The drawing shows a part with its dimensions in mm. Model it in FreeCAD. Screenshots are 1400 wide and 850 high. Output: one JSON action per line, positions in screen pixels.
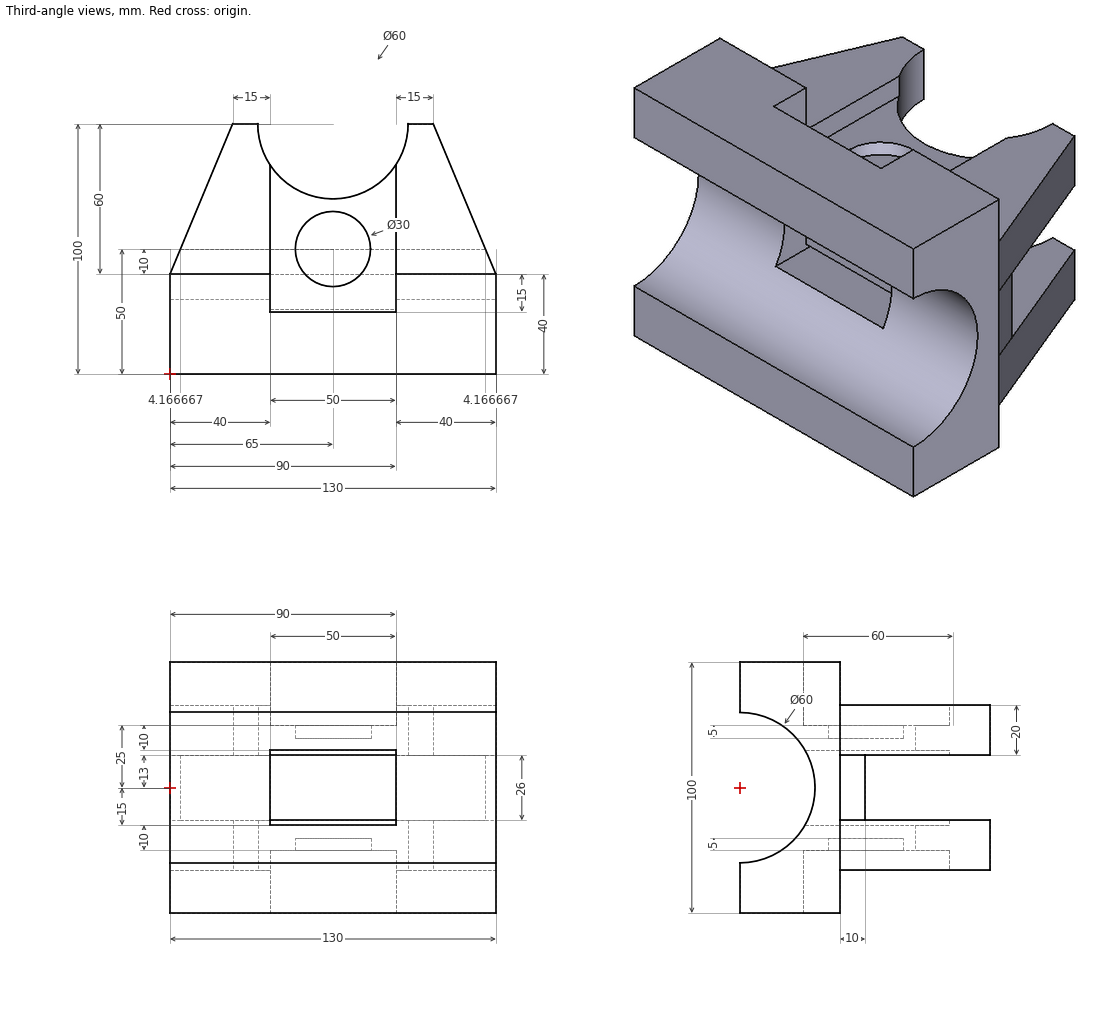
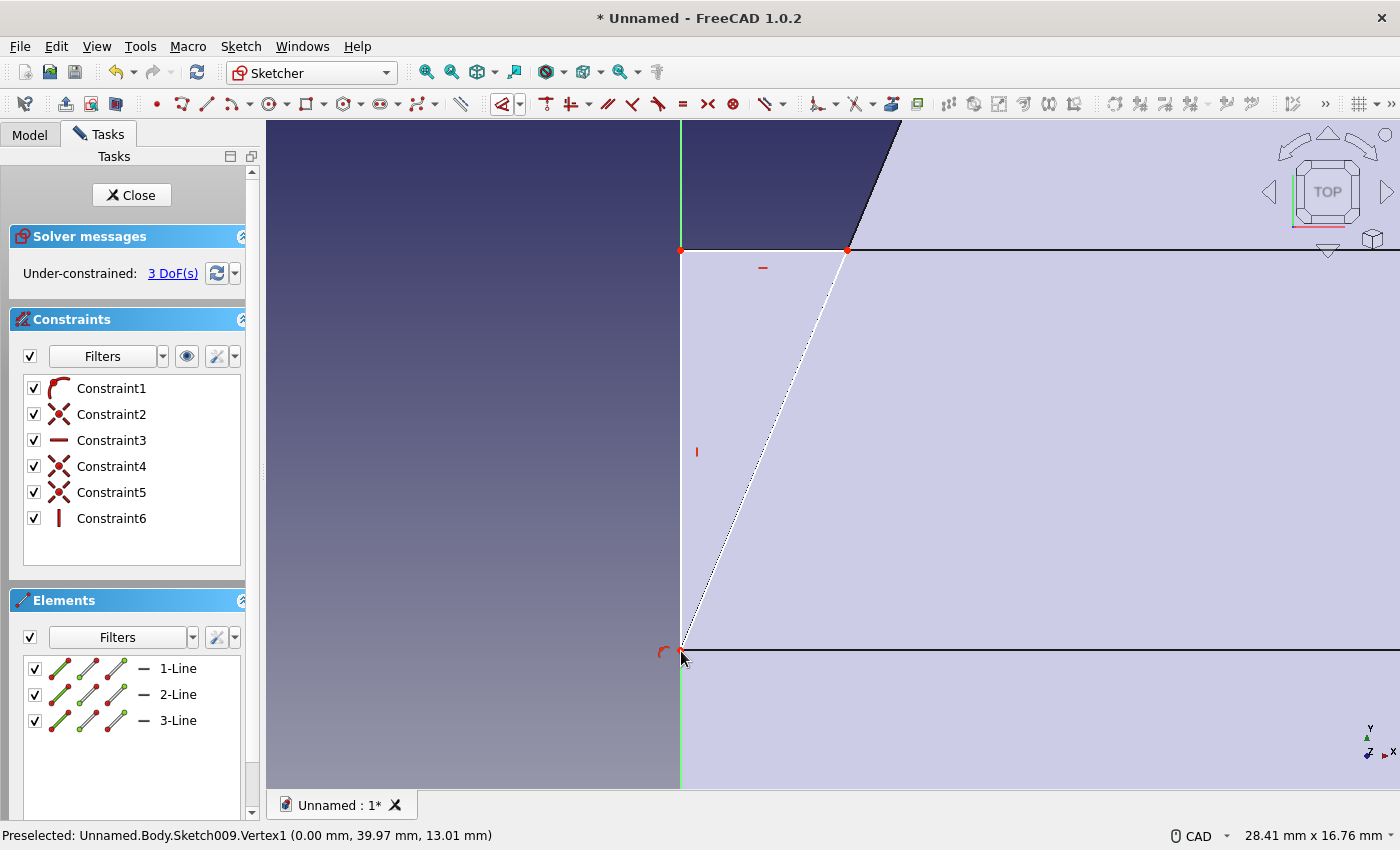
{"action": "left_click", "coordinate": [681, 371]}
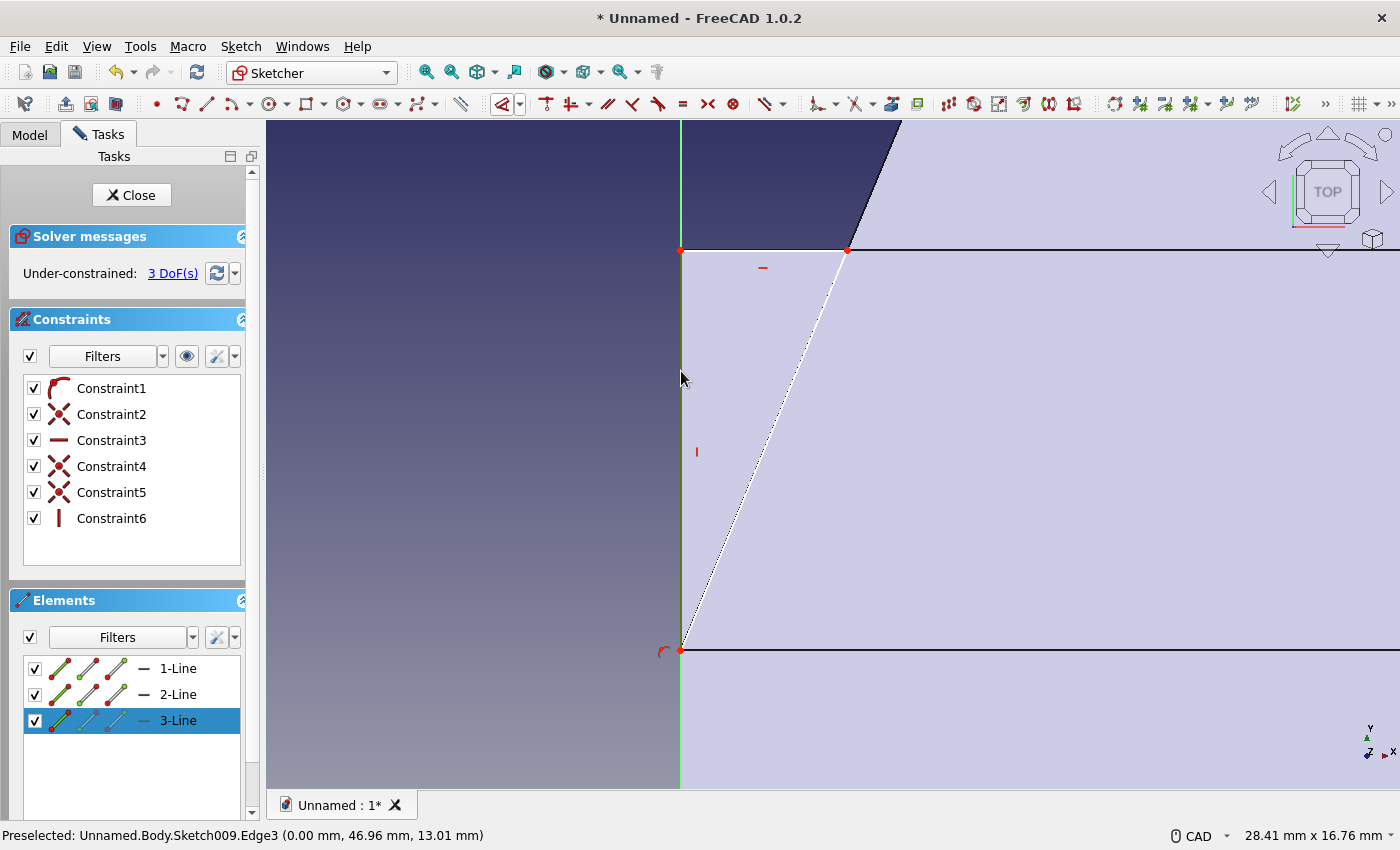
{"action": "key", "text": "i"}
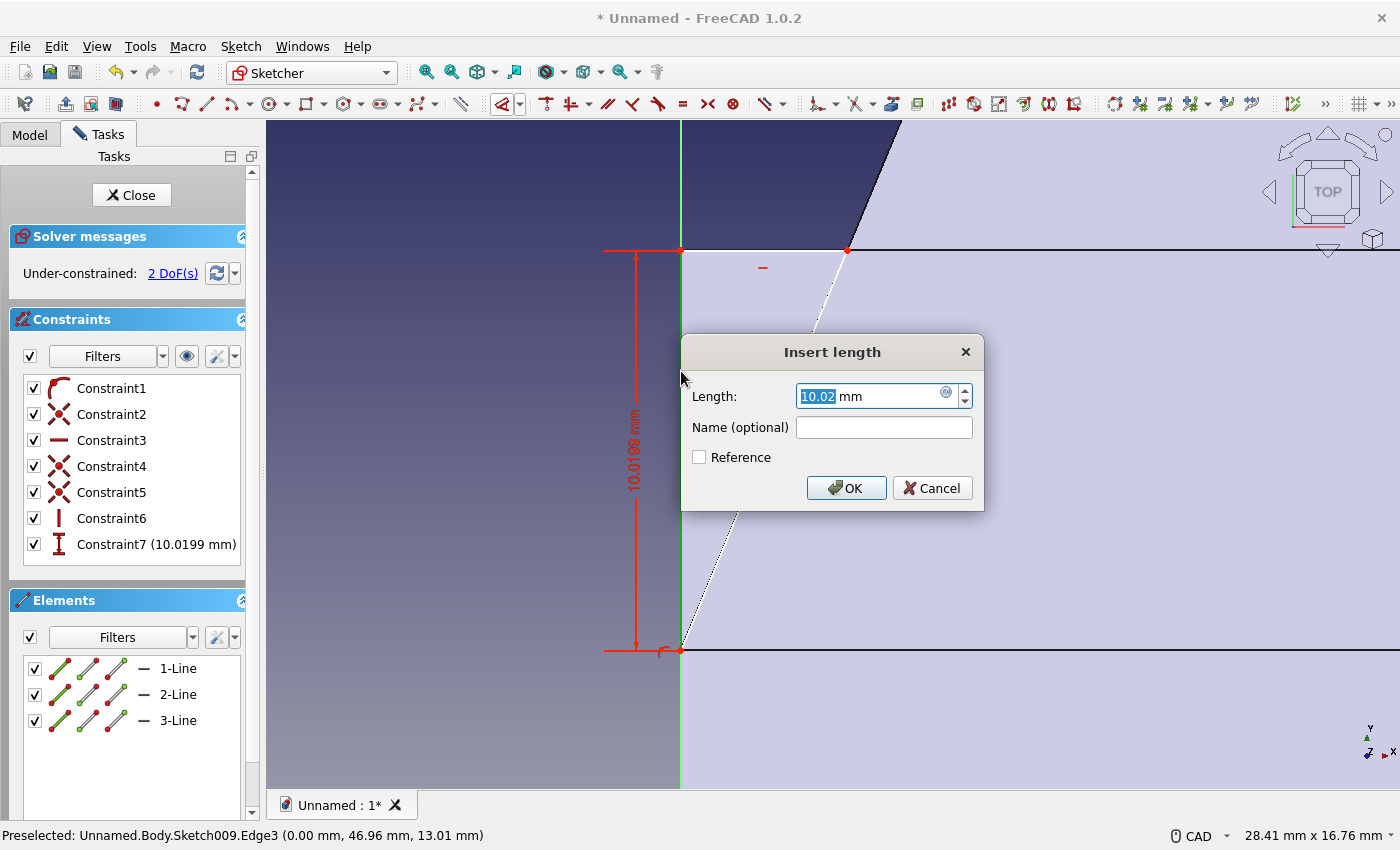
{"action": "type", "text": "10"}
{"action": "key", "text": "Return"}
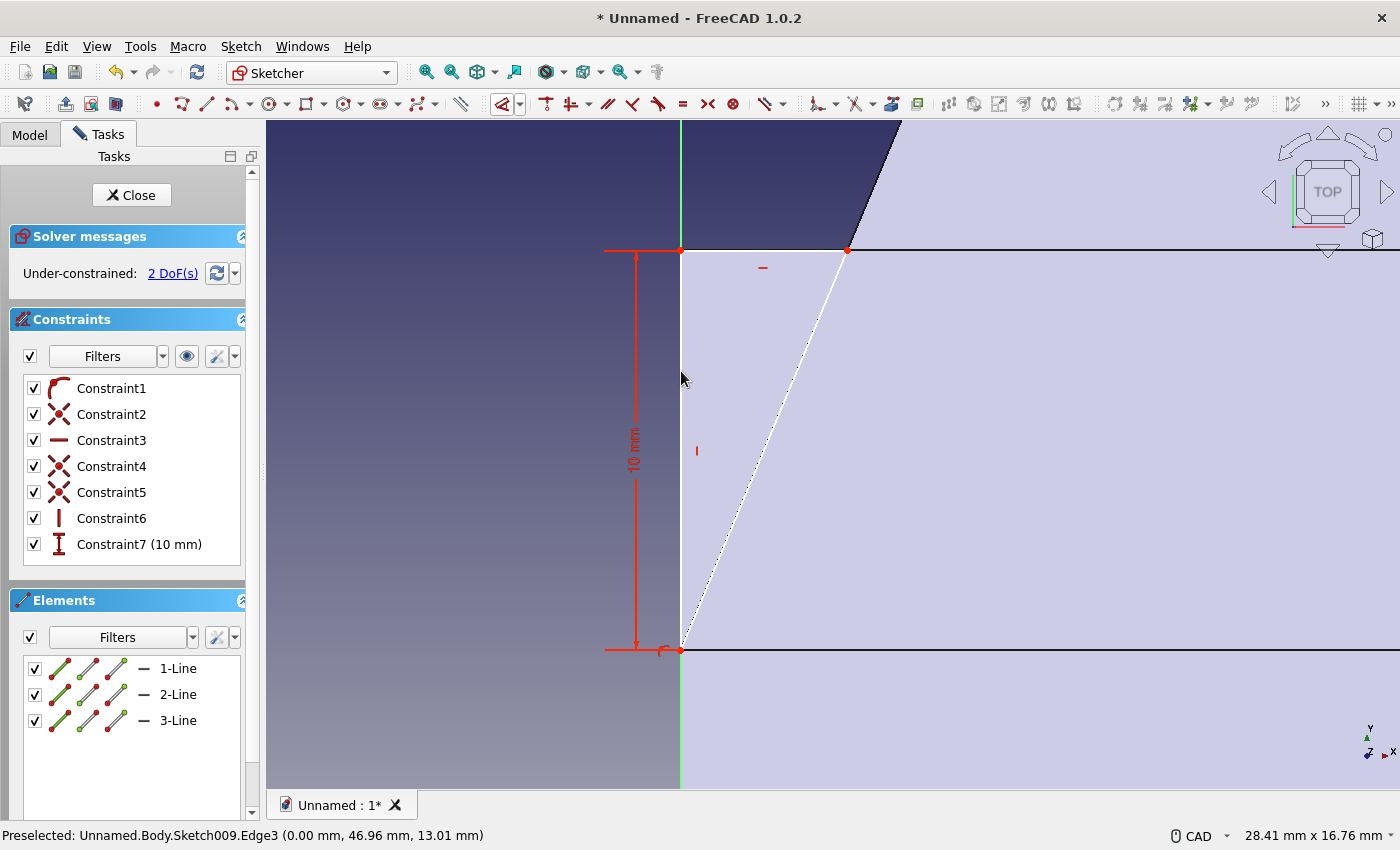
{"action": "left_click", "coordinate": [681, 650]}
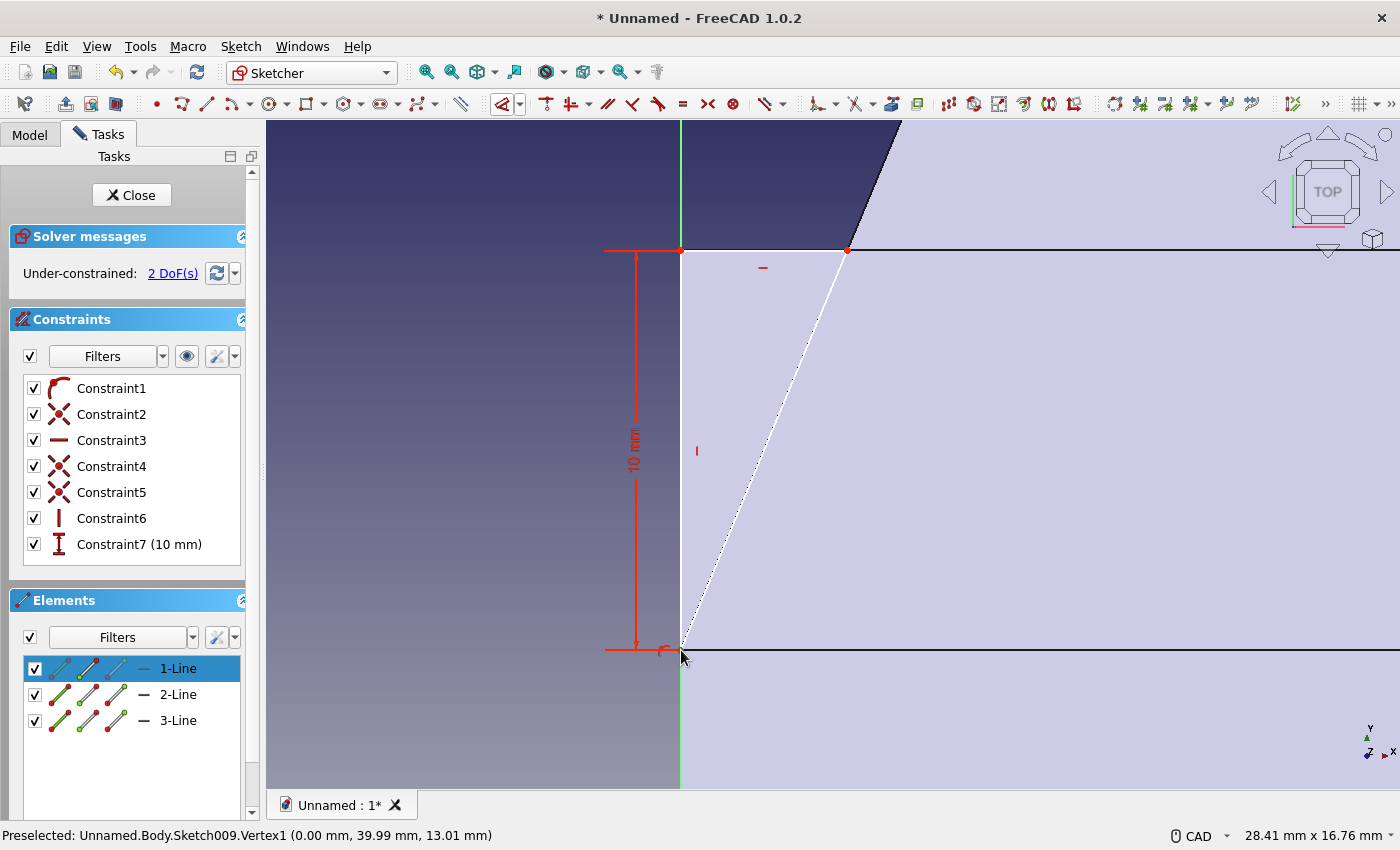
{"action": "left_click", "coordinate": [520, 104]}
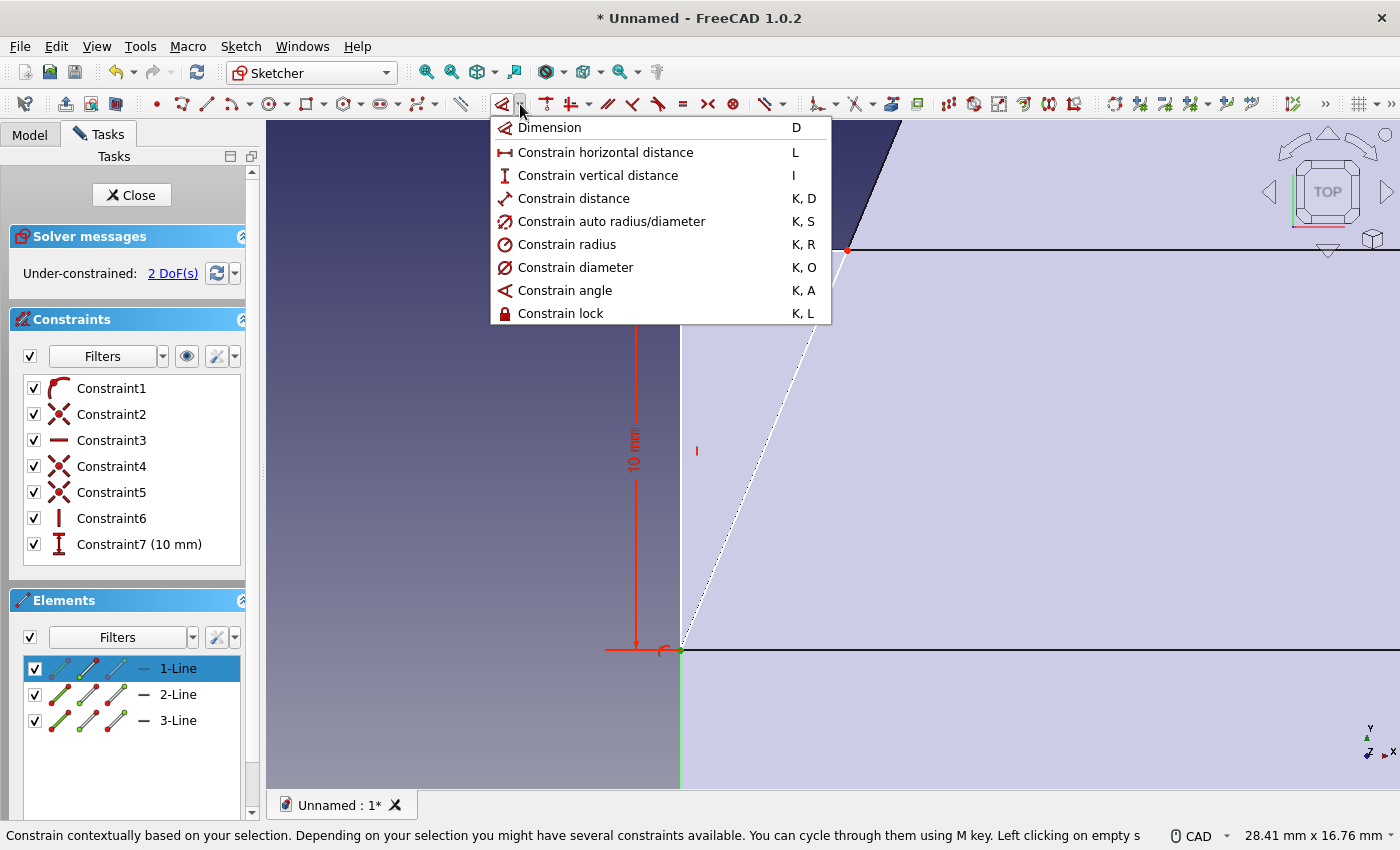
{"action": "left_click", "coordinate": [661, 176]}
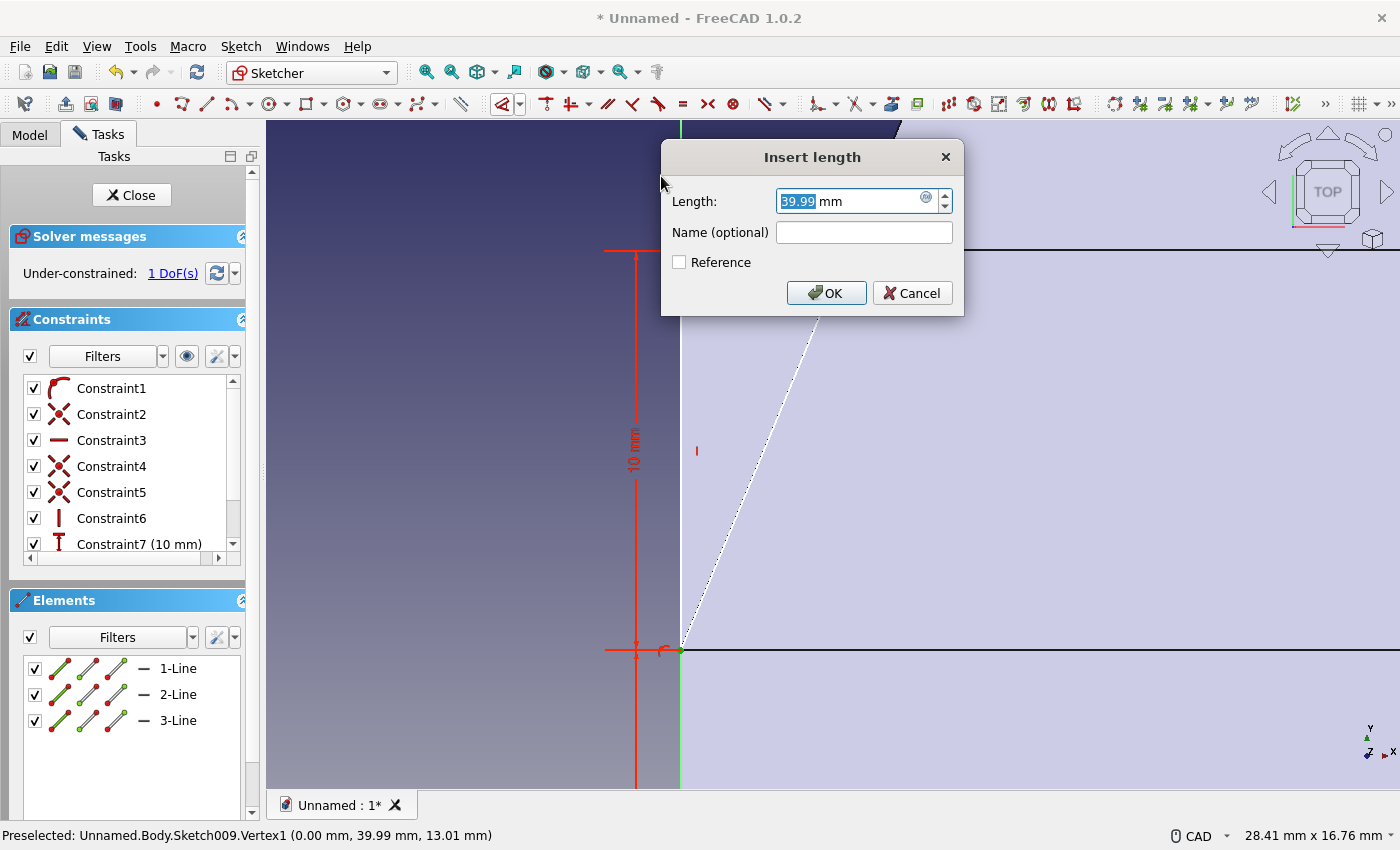
{"action": "type", "text": "40"}
{"action": "key", "text": "Return"}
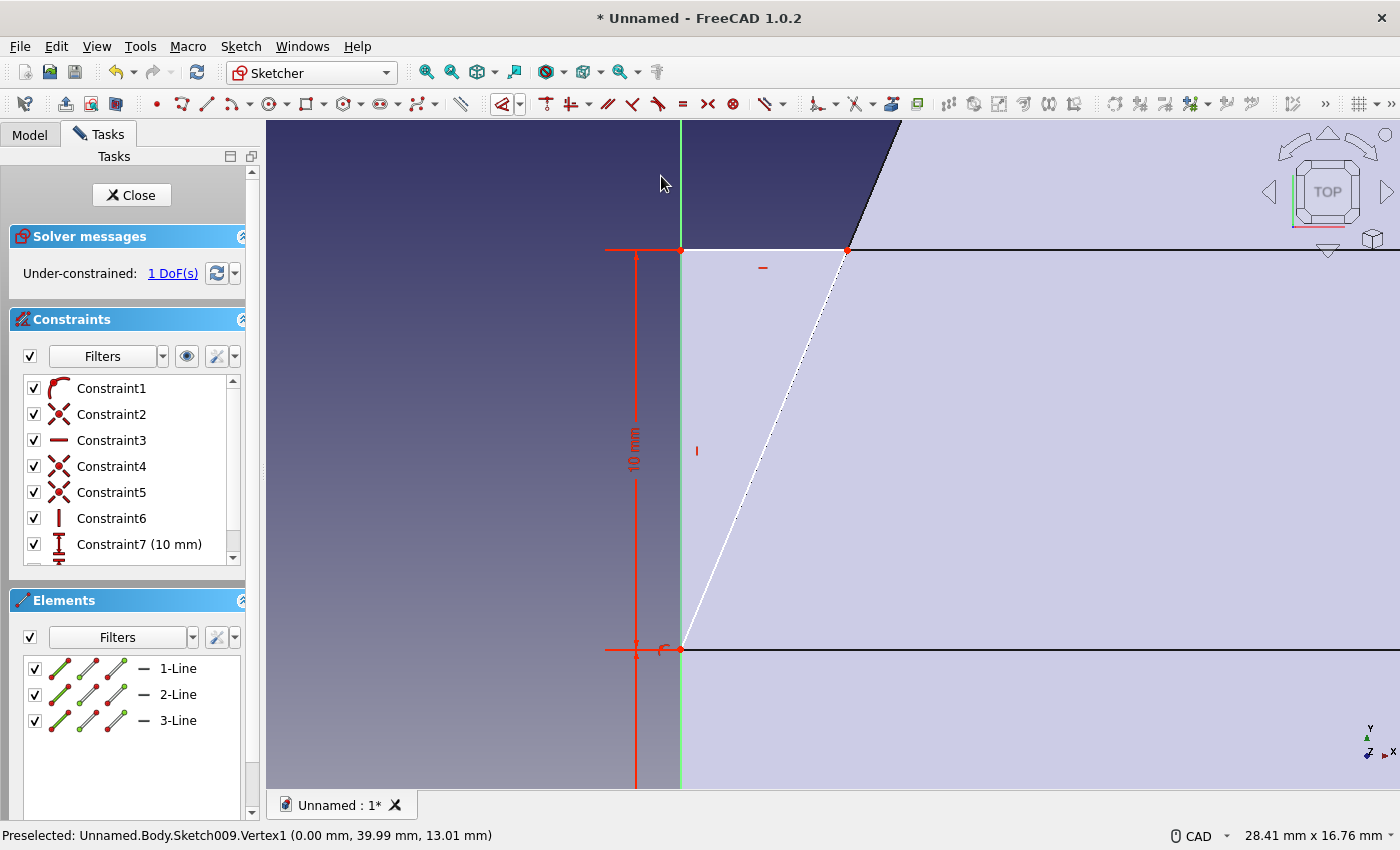
{"action": "left_click", "coordinate": [797, 250]}